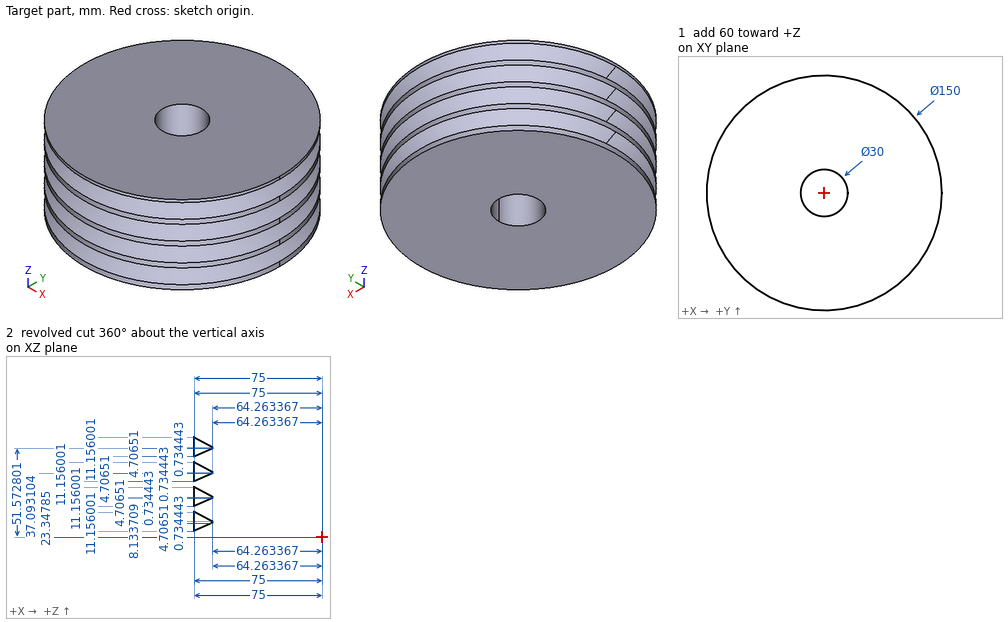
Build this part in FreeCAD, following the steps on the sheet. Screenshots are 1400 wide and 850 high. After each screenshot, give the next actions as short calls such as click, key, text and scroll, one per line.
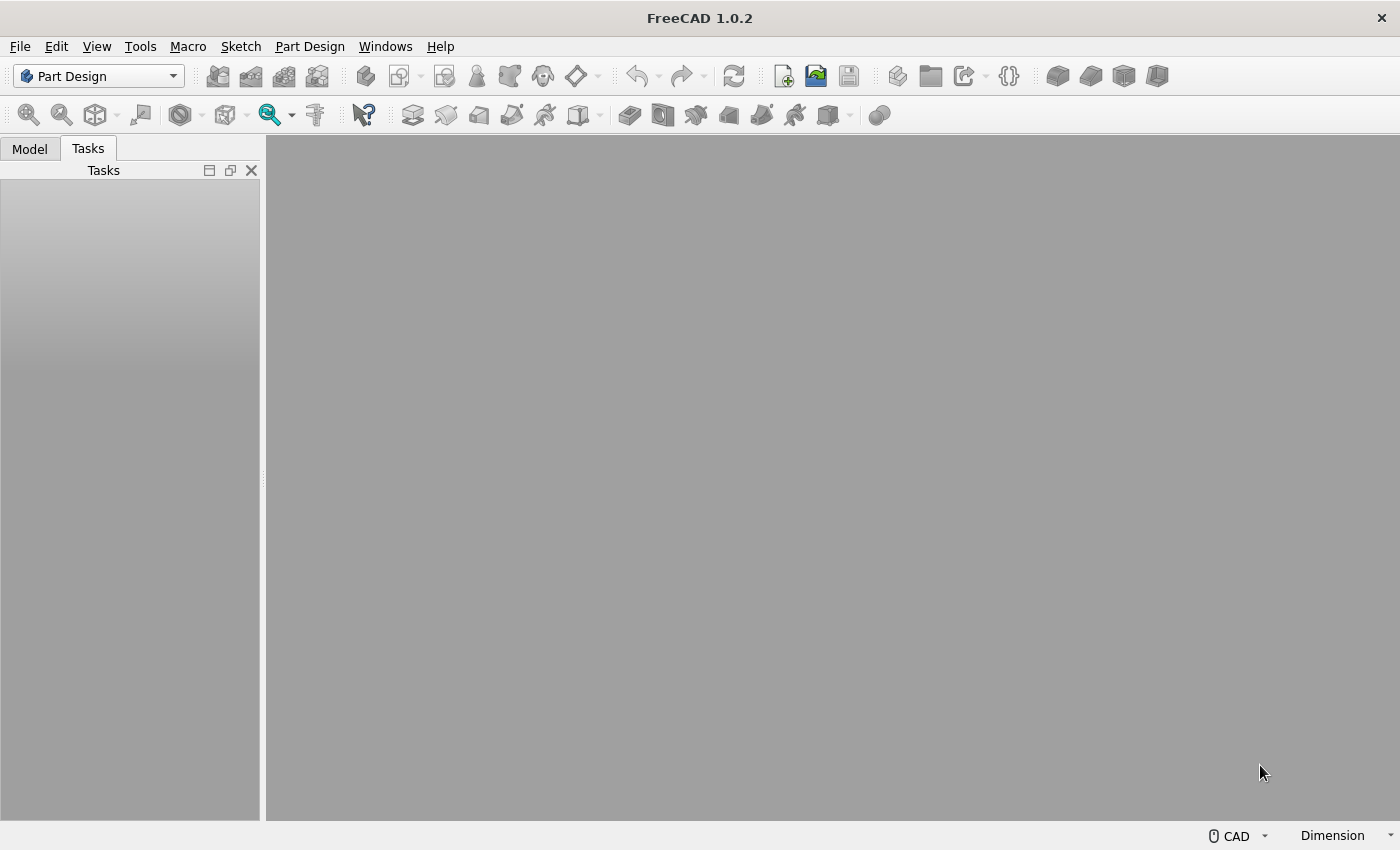
click(783, 76)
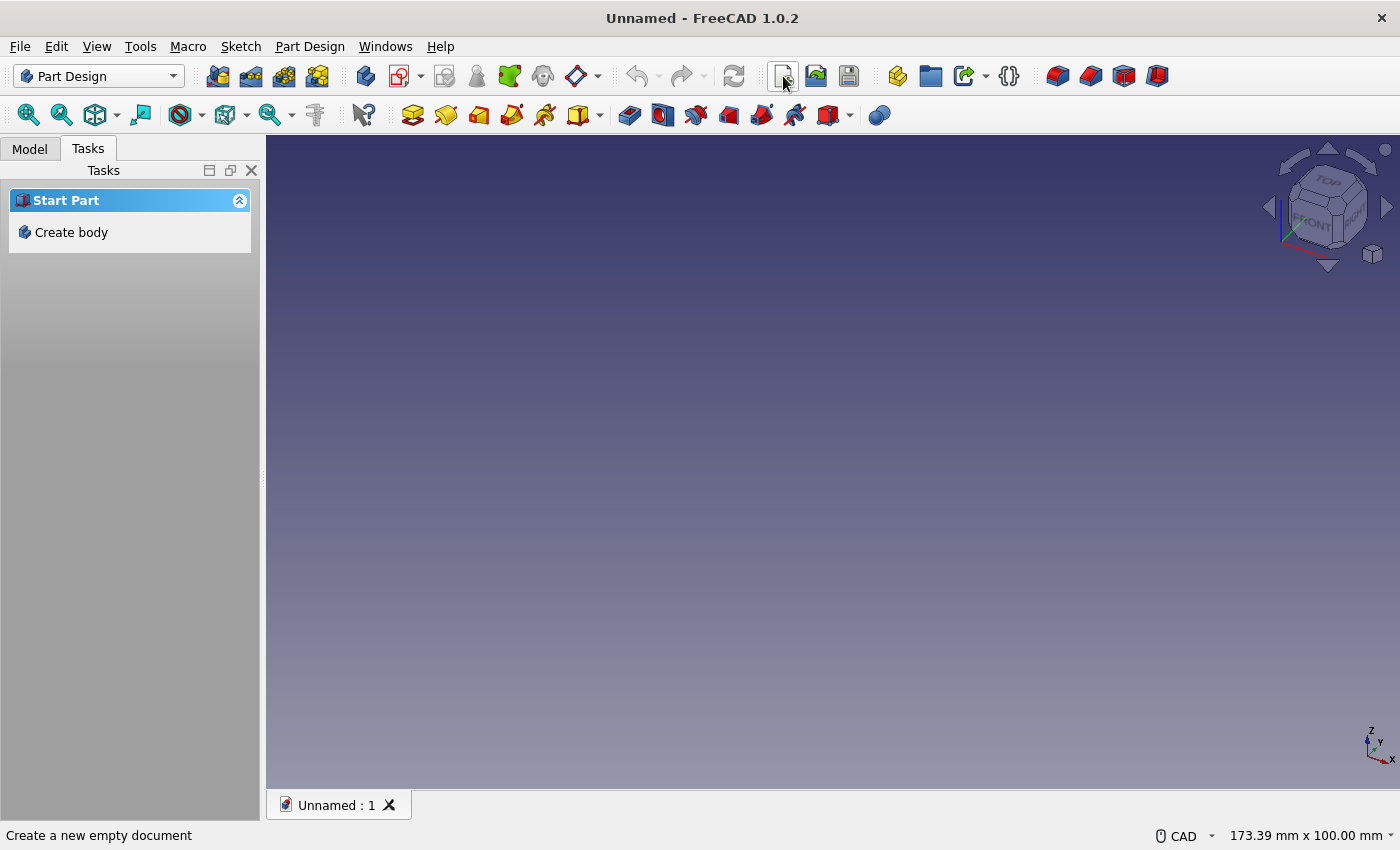
click(398, 76)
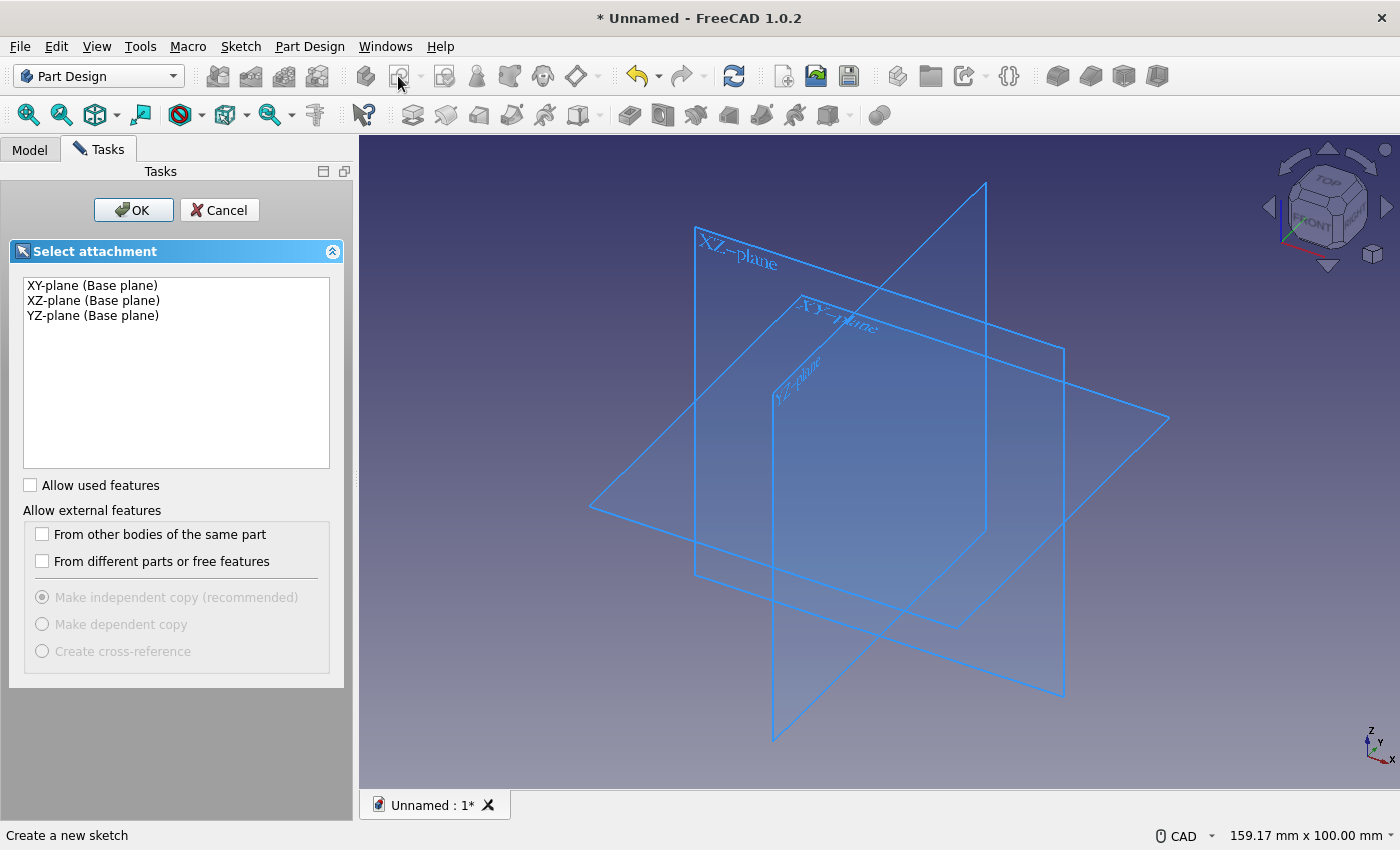
click(84, 286)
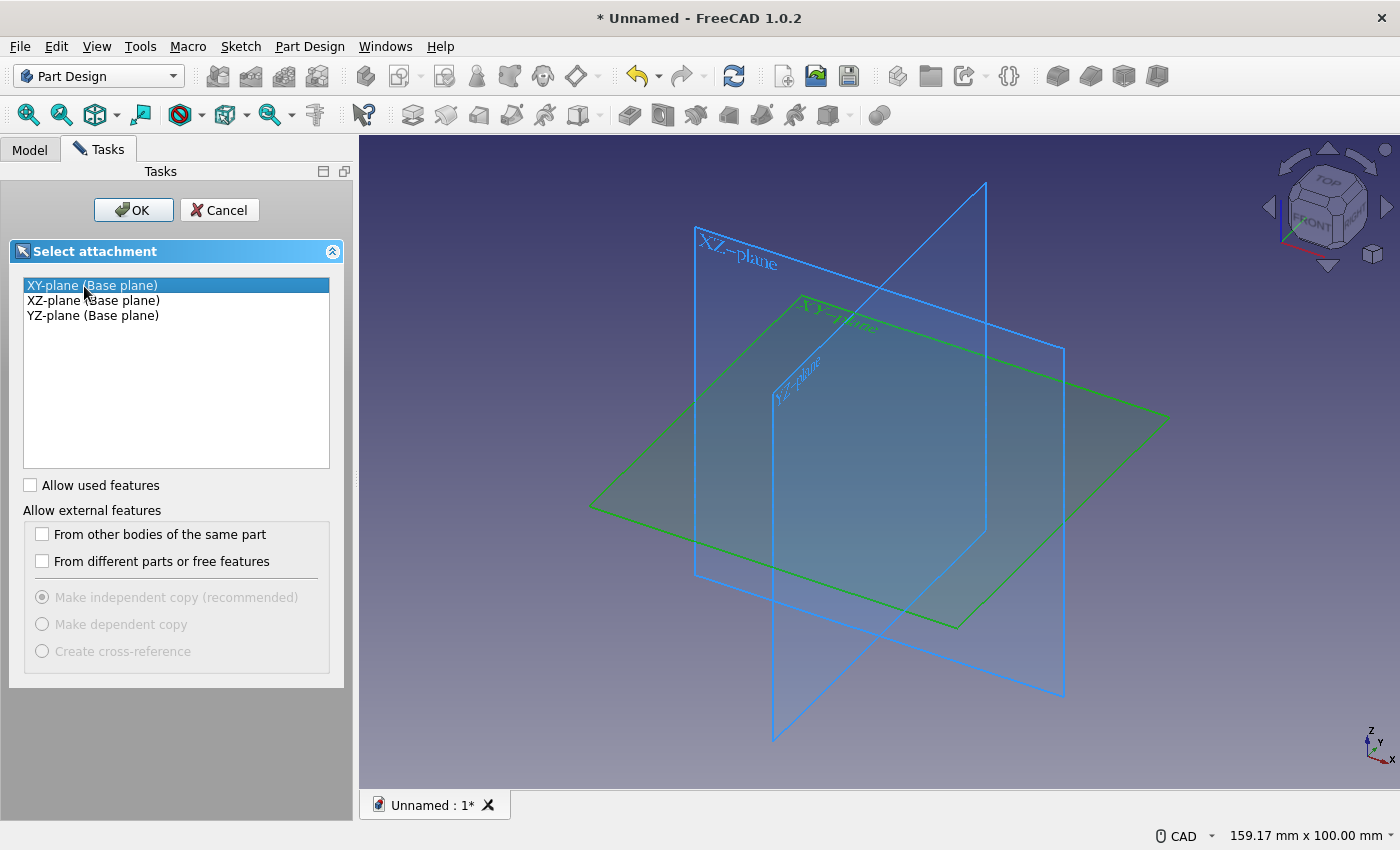
click(134, 210)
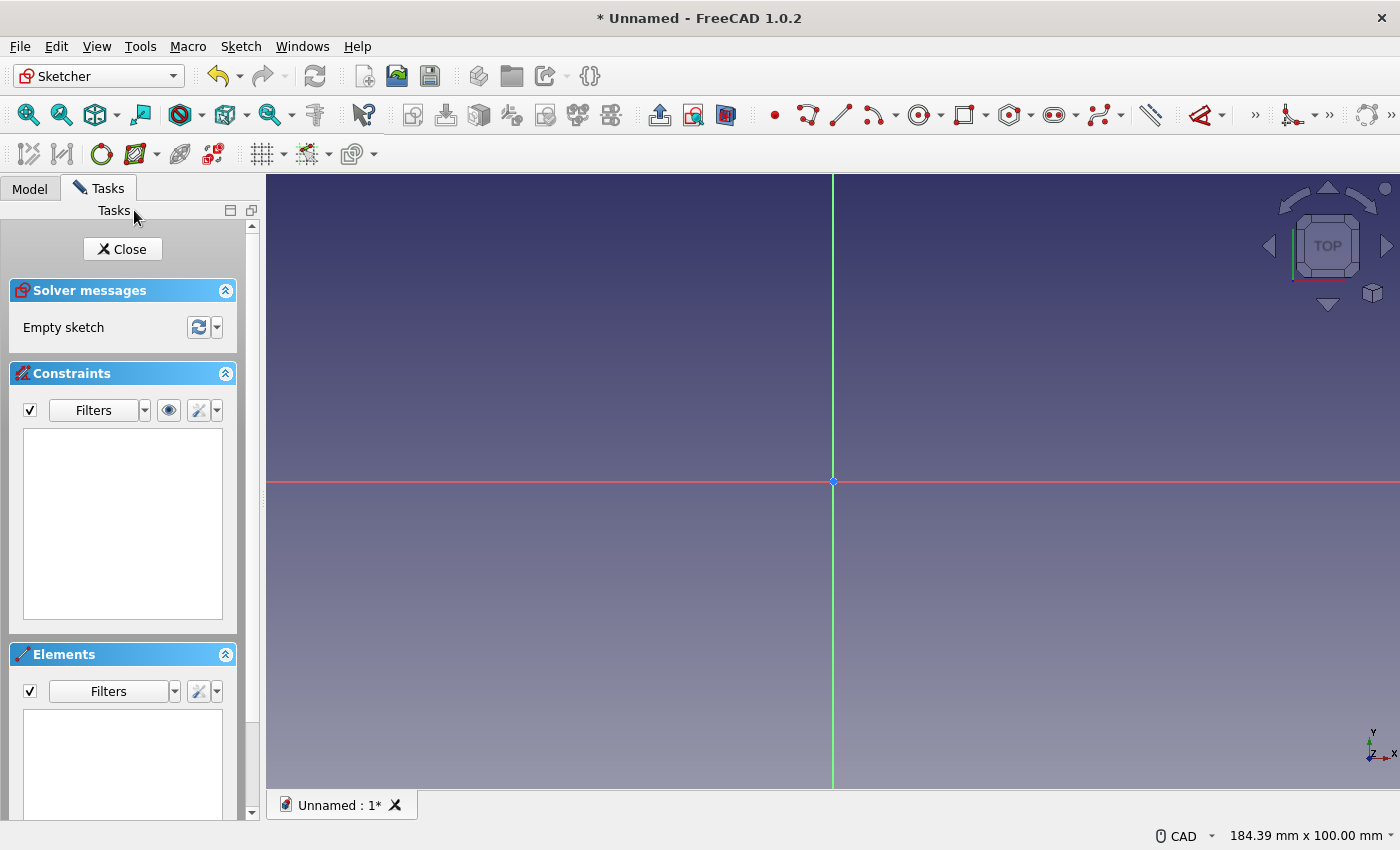
scroll(709, 482, down, 4)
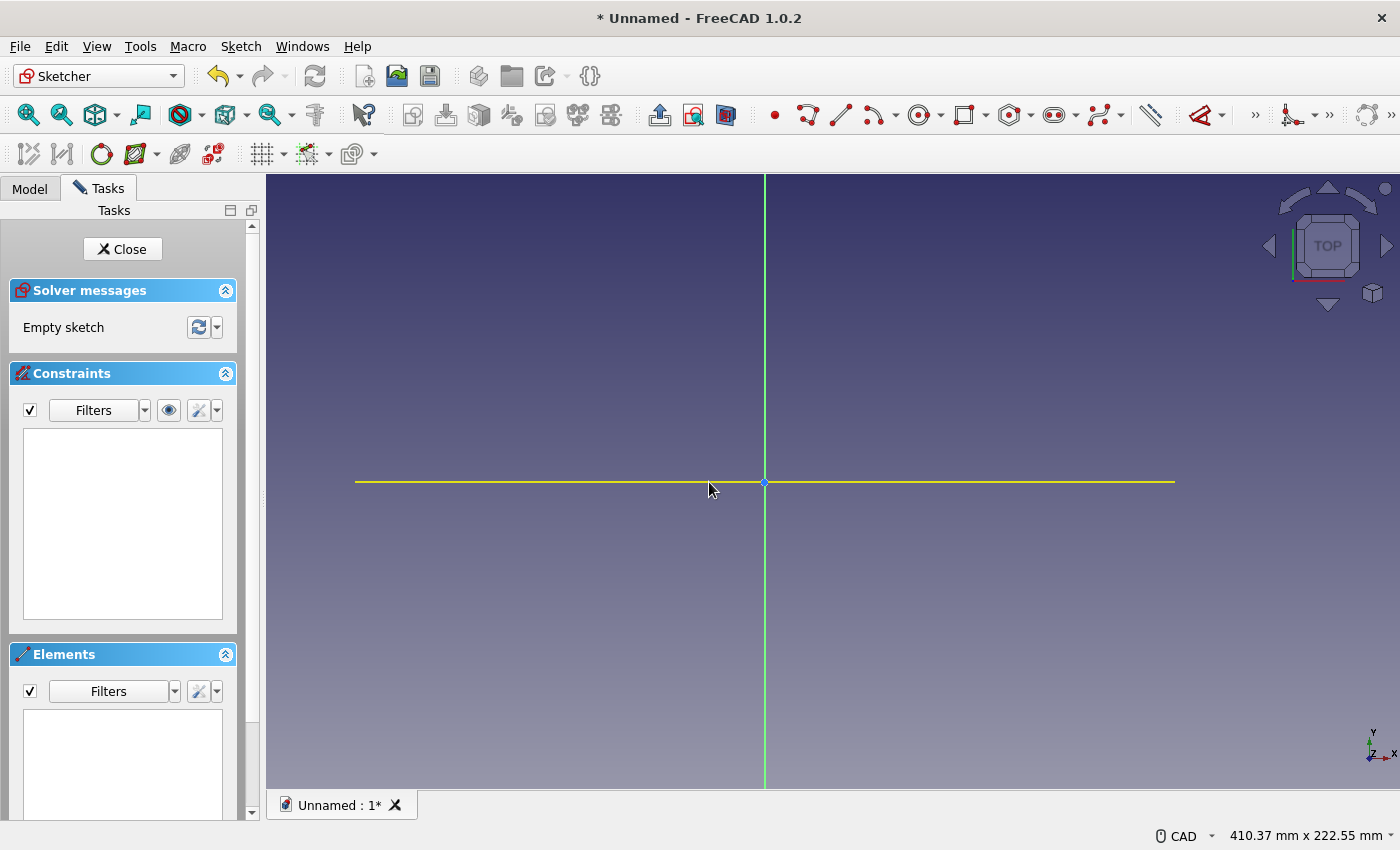
click(918, 116)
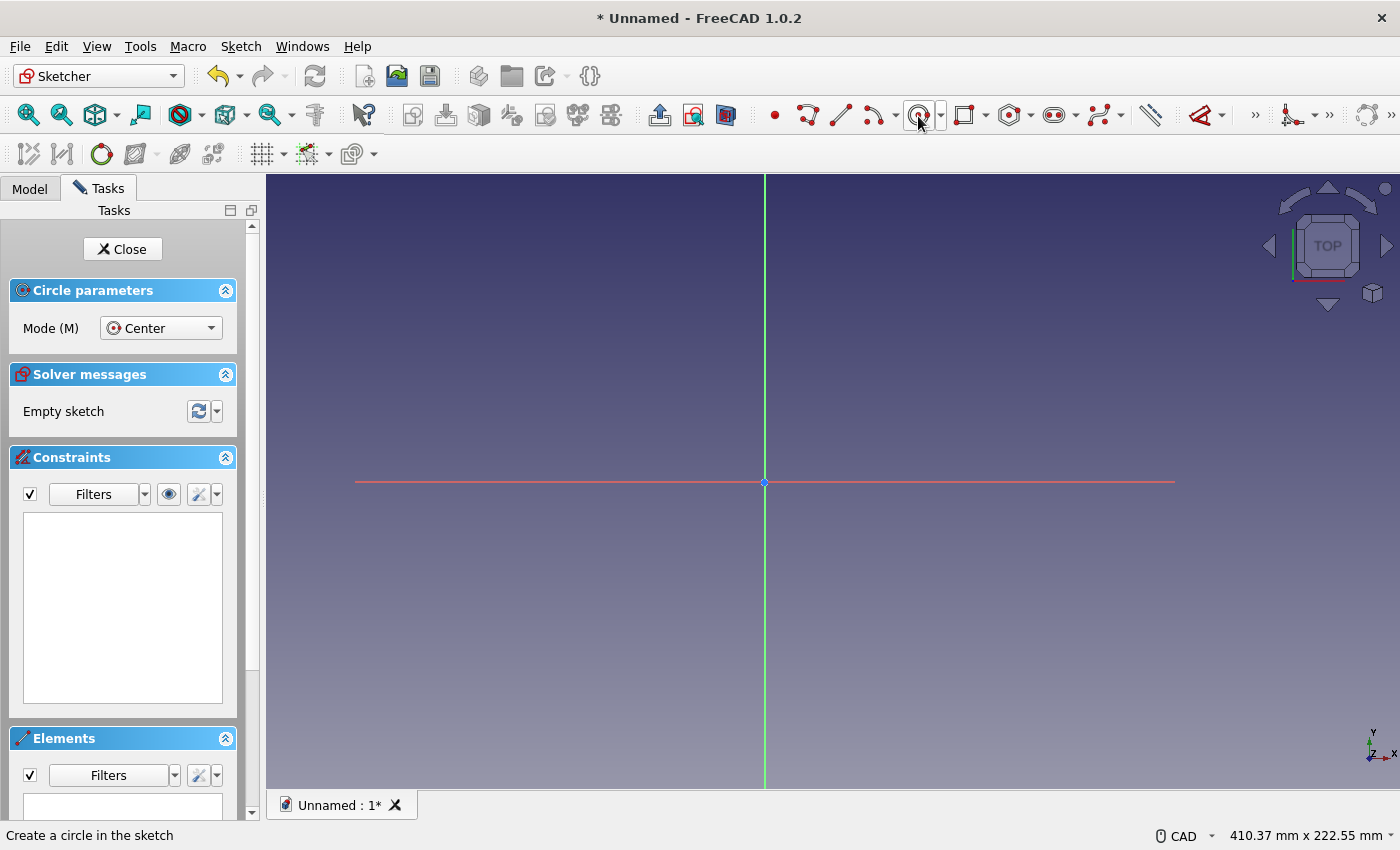
click(765, 482)
move(911, 336)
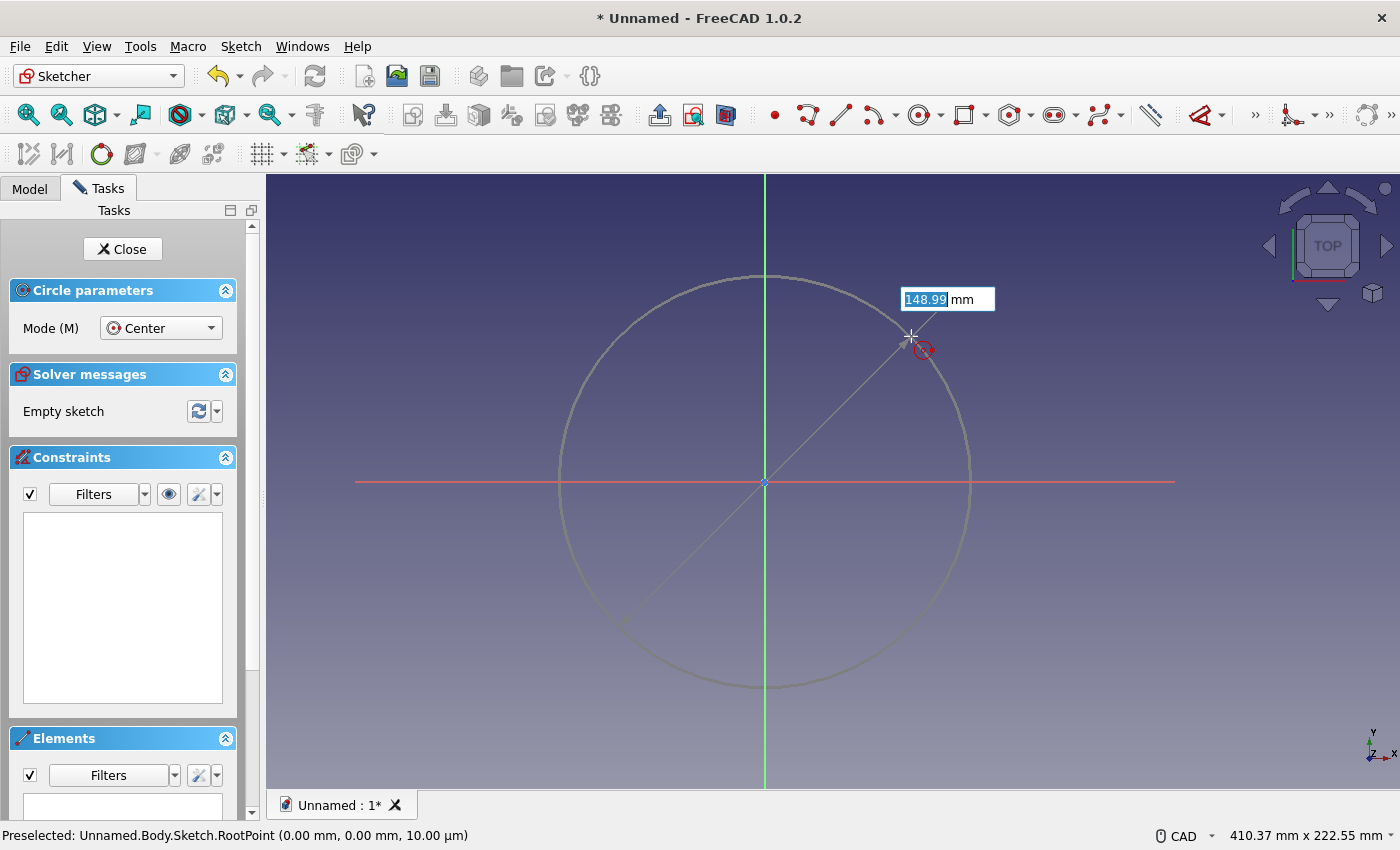
text(150)
key(Return)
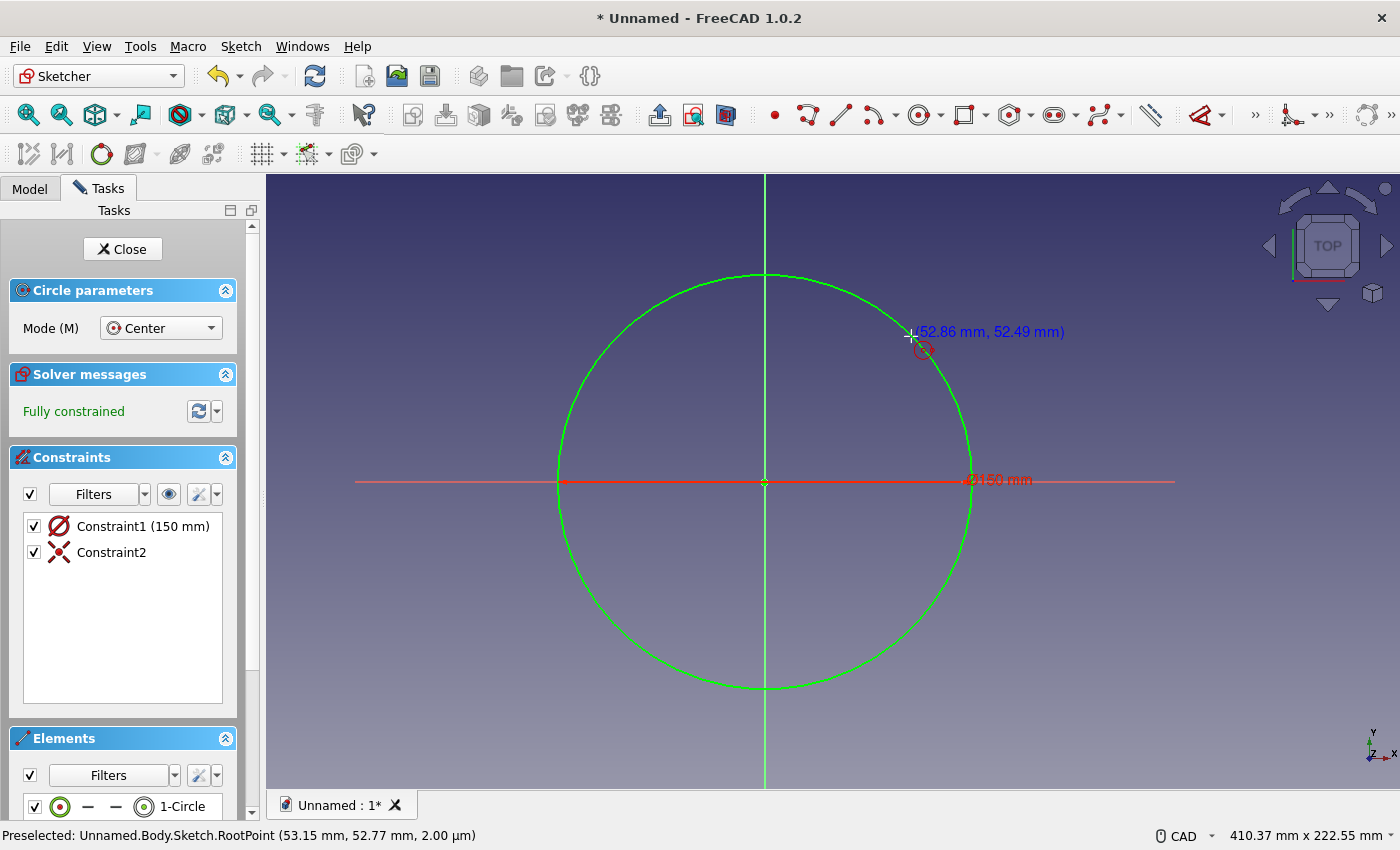
click(765, 482)
move(794, 453)